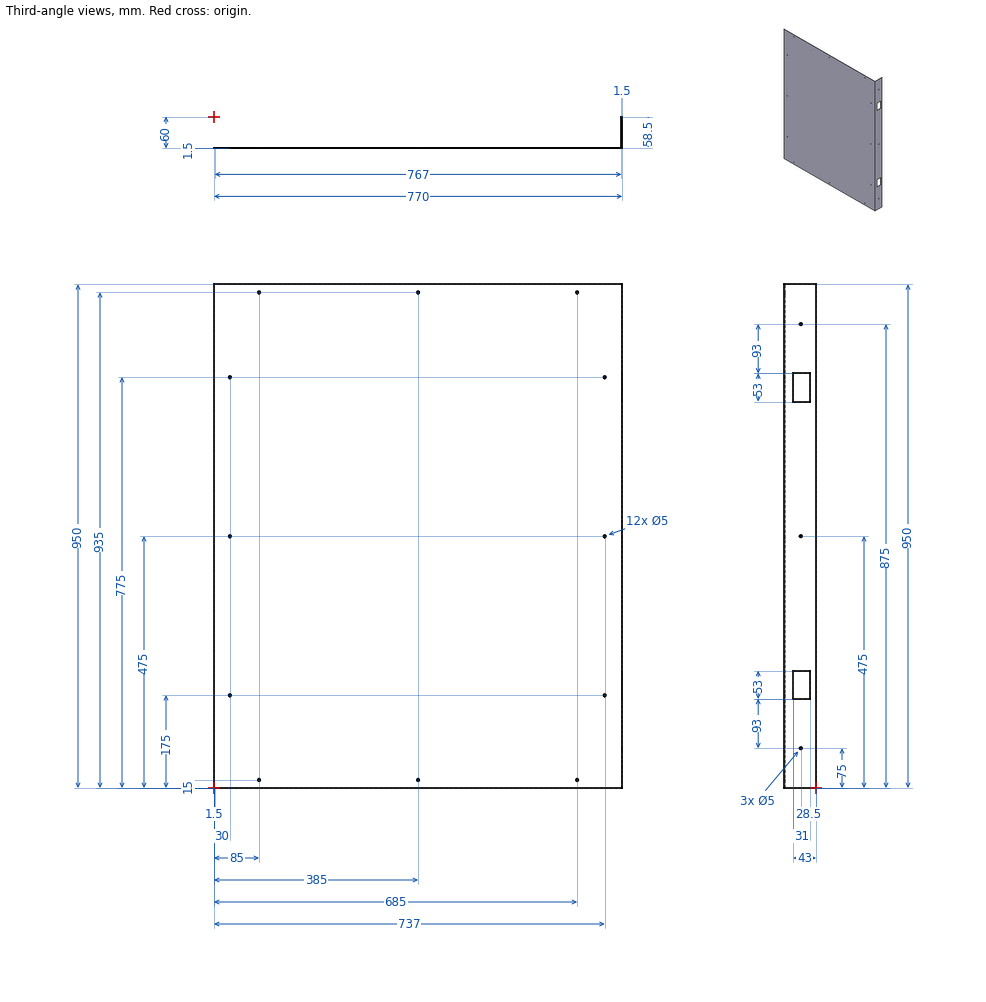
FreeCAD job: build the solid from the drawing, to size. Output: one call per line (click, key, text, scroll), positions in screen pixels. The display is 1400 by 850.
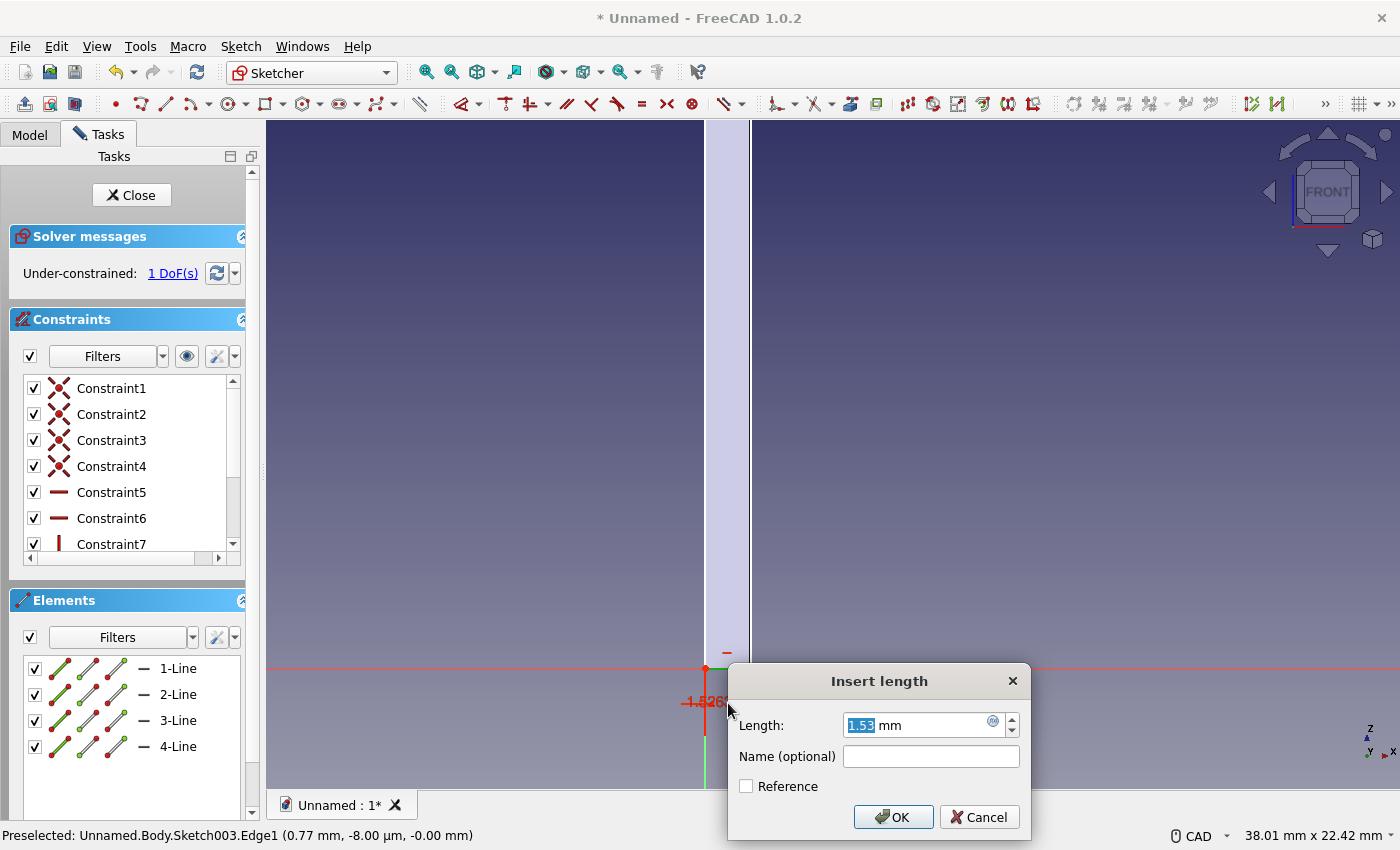
text(1.5)
key(Return)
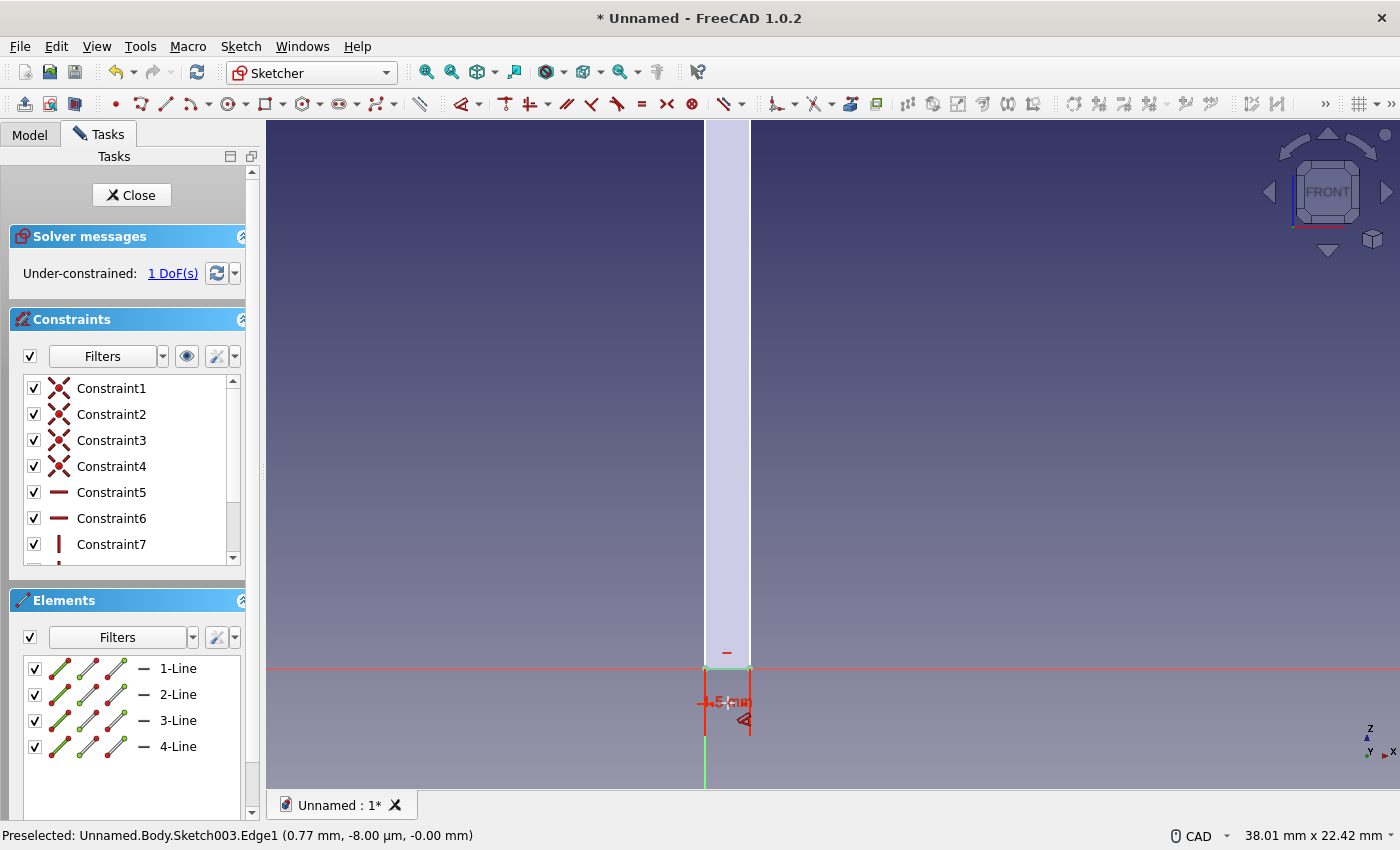
scroll(764, 454, down, 15)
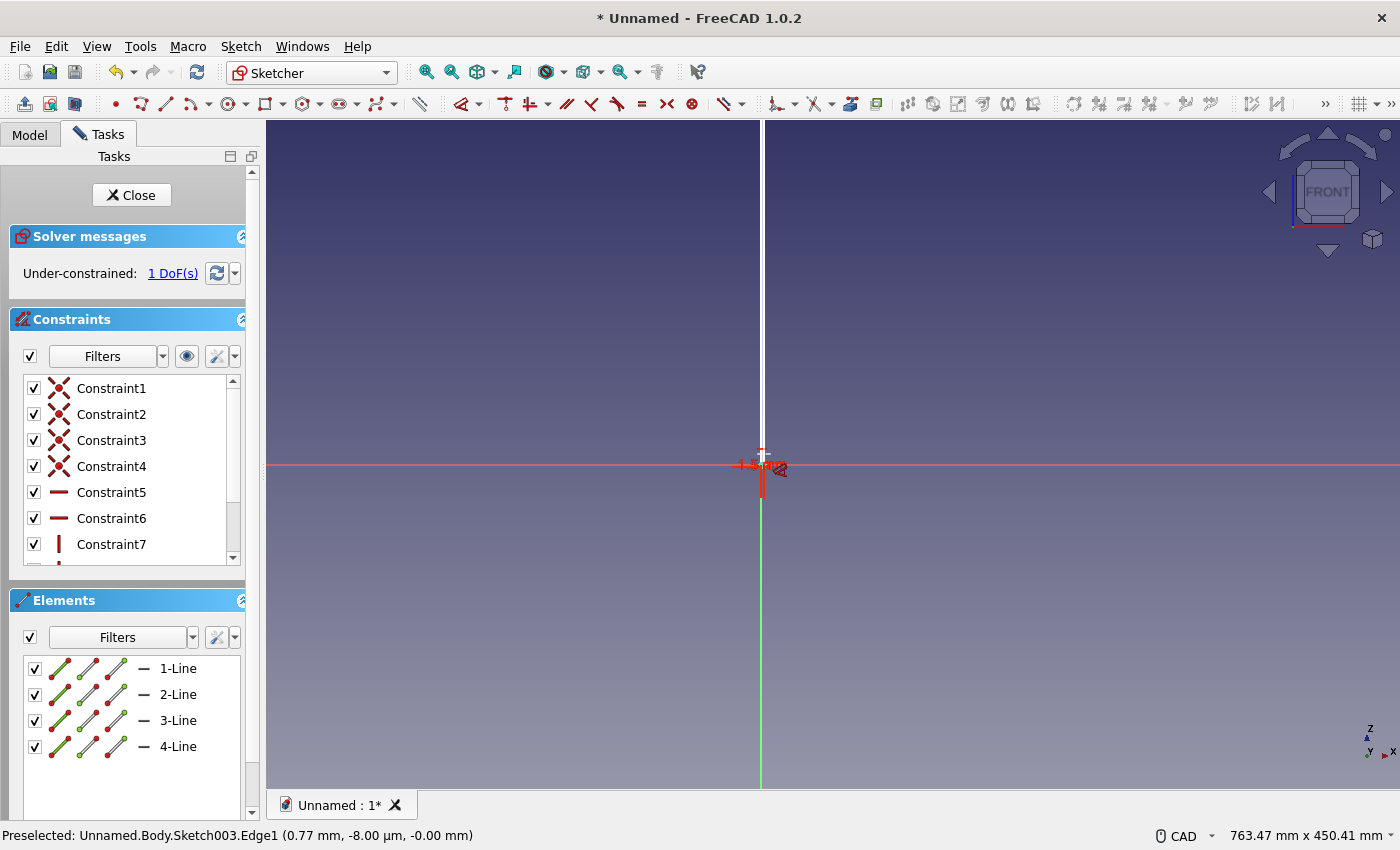
scroll(765, 754, down, 6)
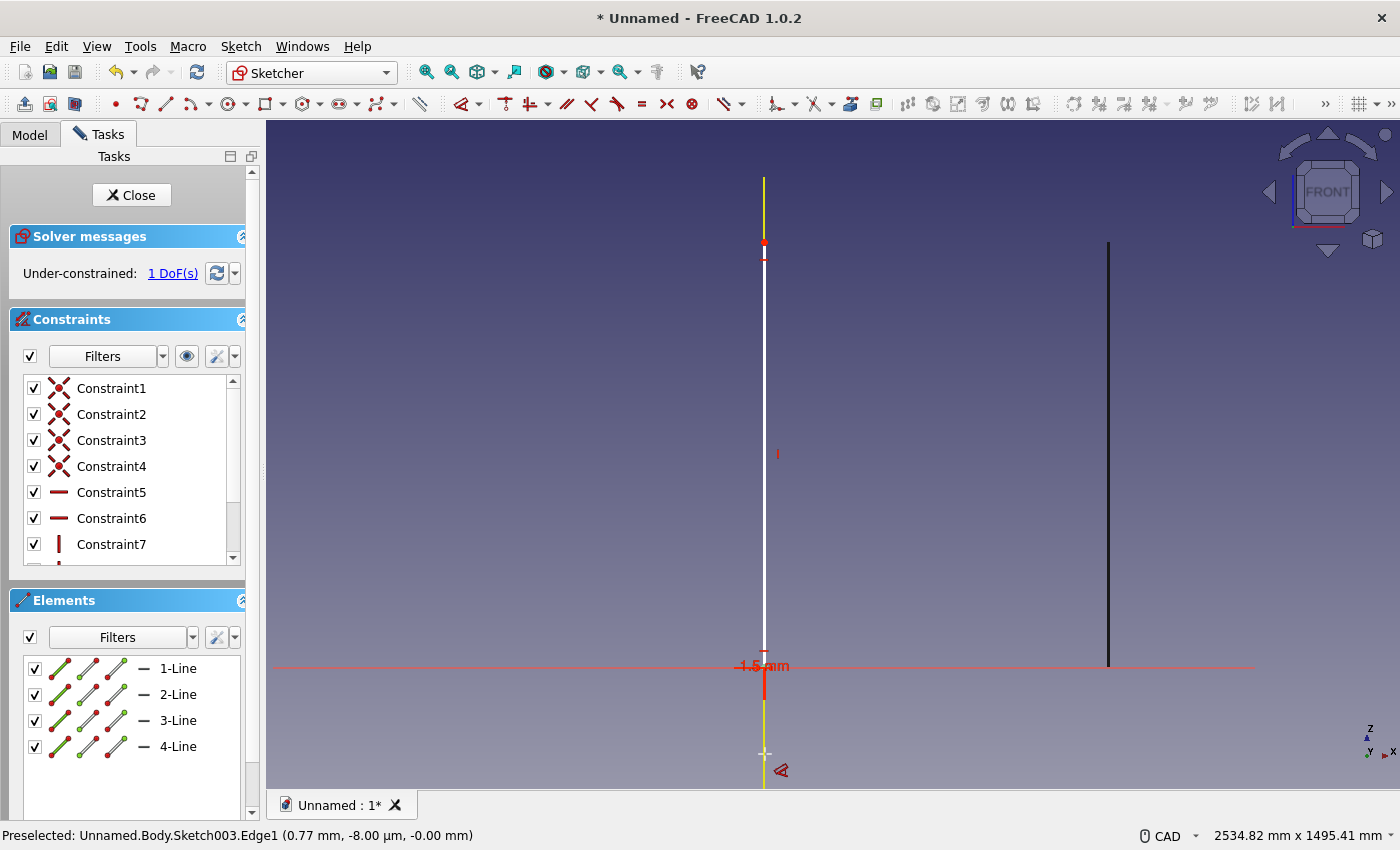
scroll(765, 540, up, 15)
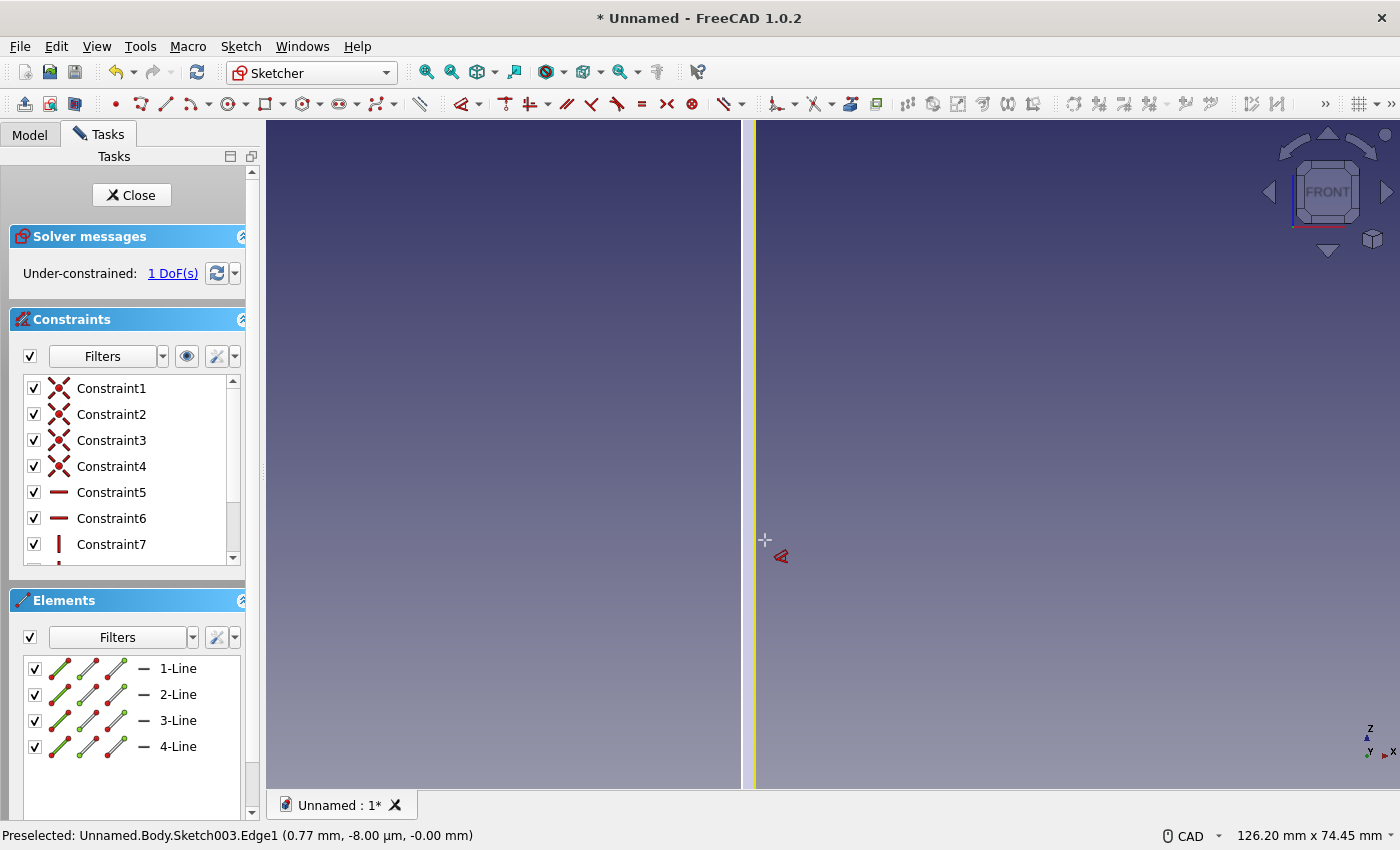
click(755, 532)
click(789, 454)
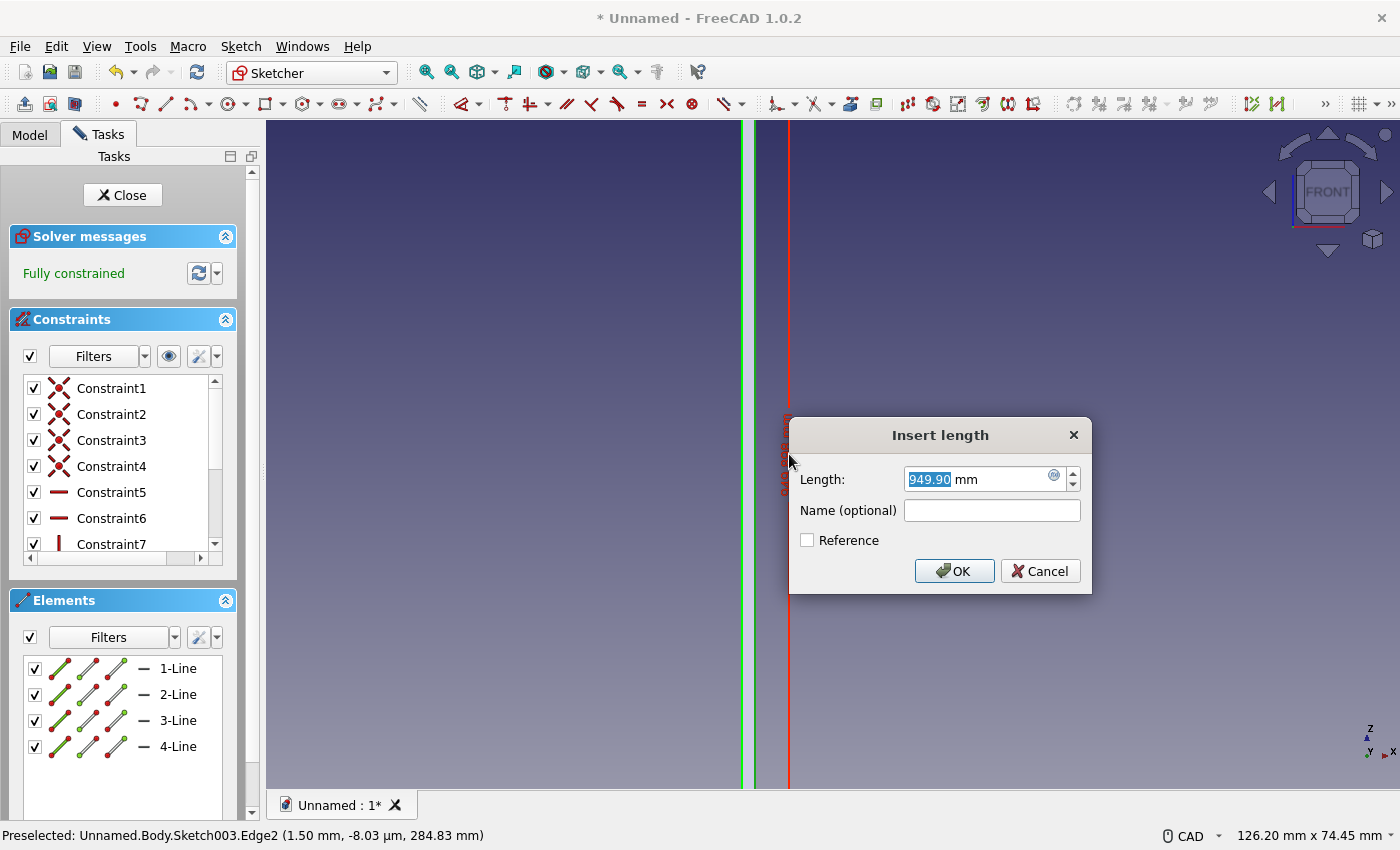
text(950)
key(Return)
key(Escape)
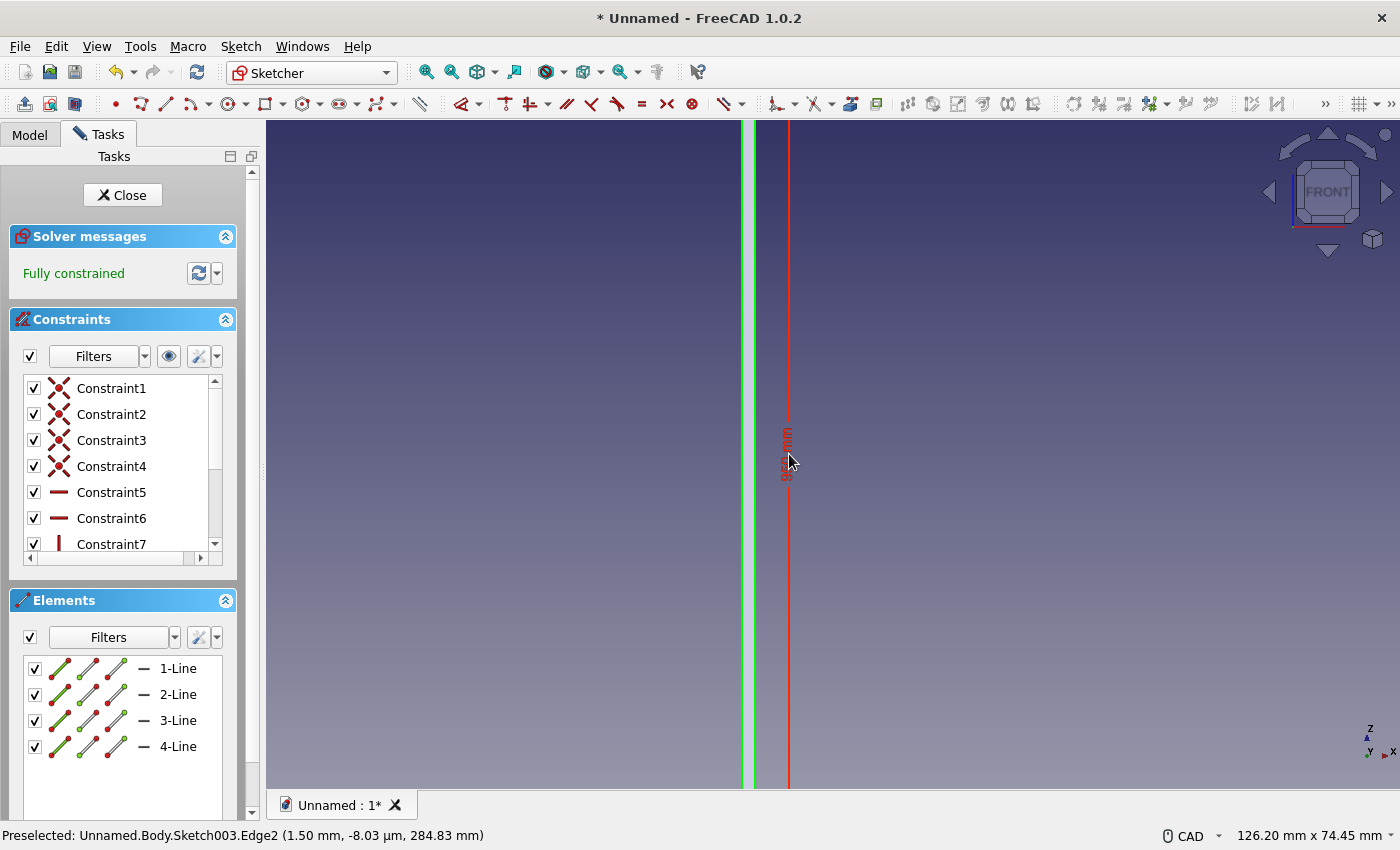
click(123, 195)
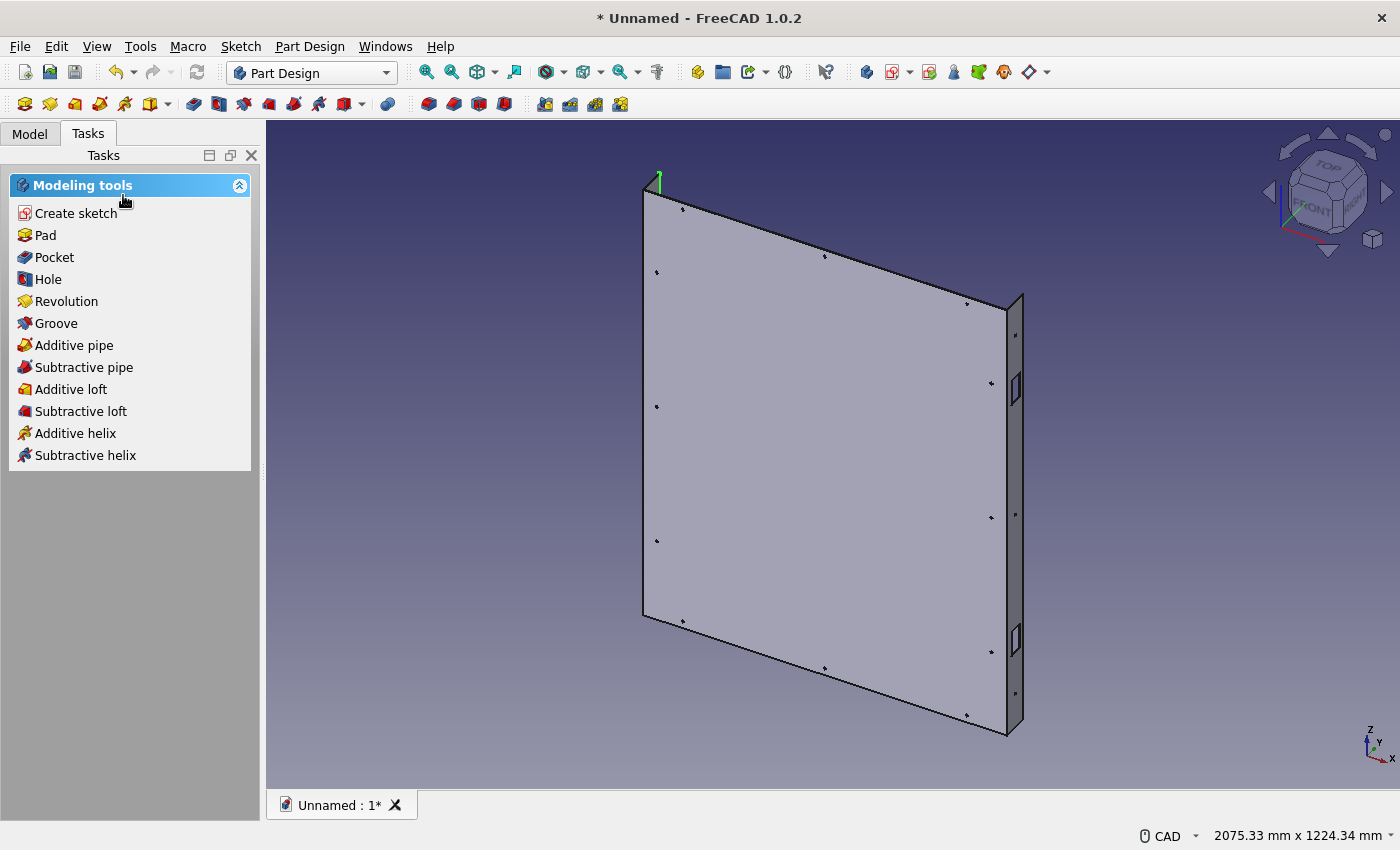
click(194, 104)